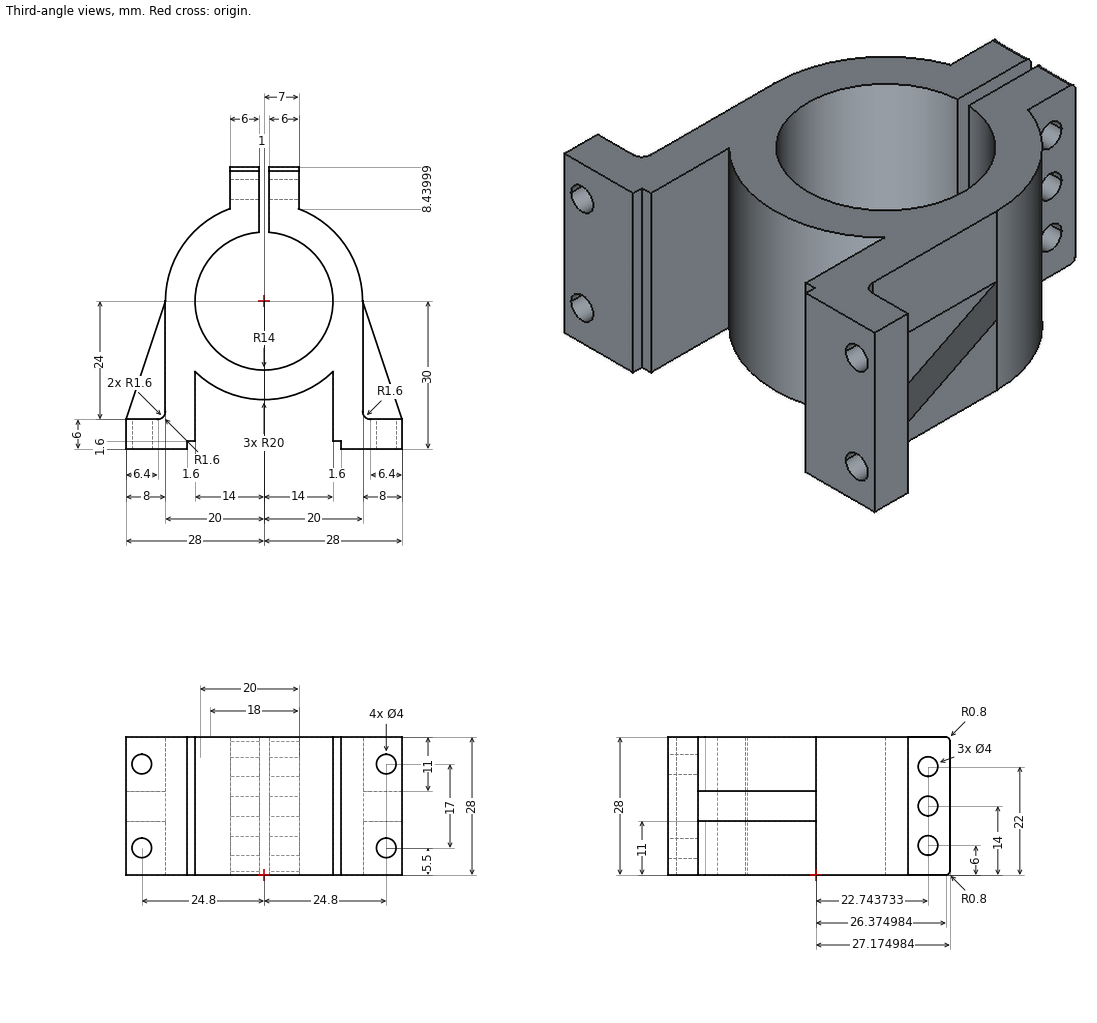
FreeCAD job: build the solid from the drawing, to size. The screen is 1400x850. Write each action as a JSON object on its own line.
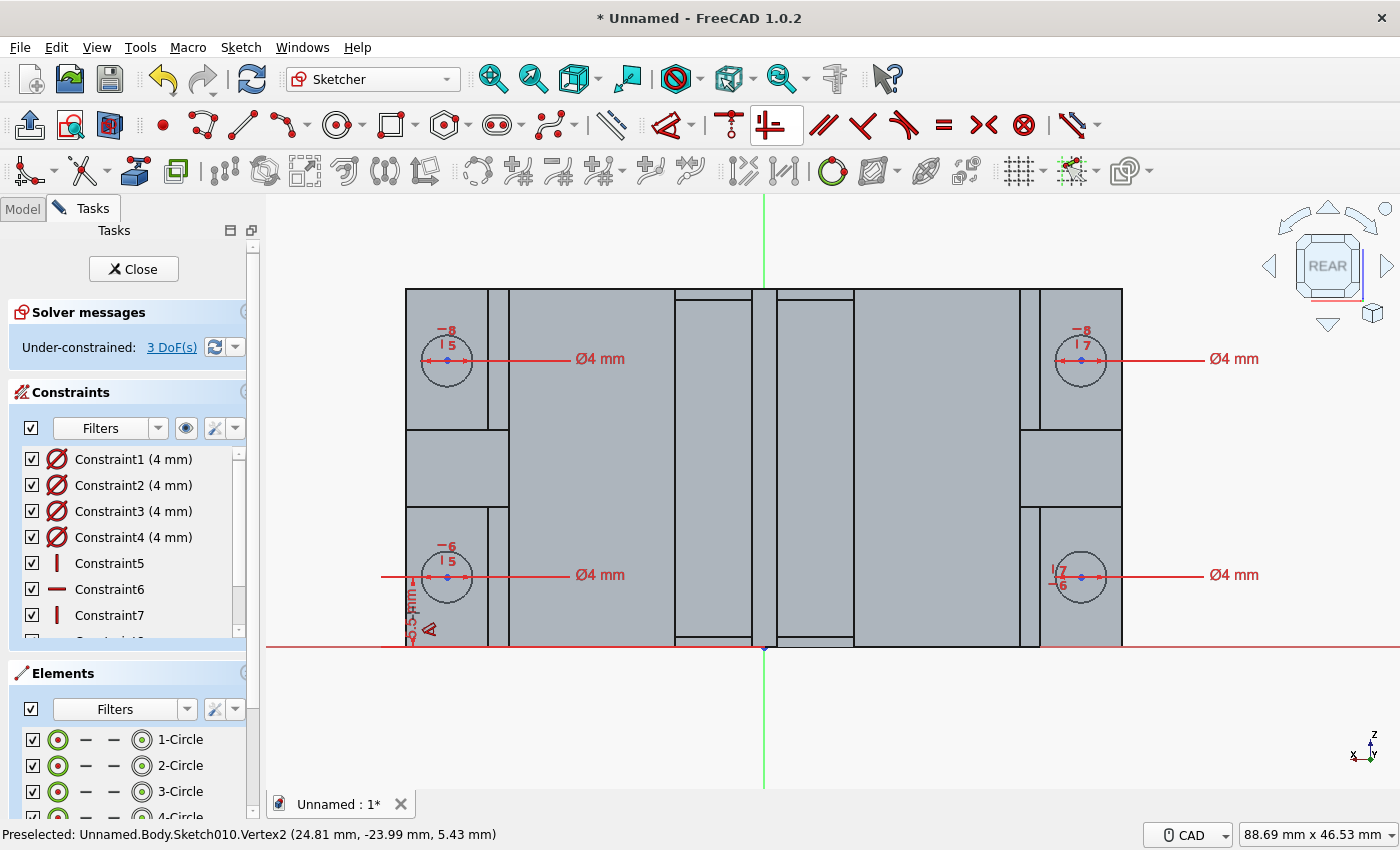
{"action": "left_click", "coordinate": [447, 361]}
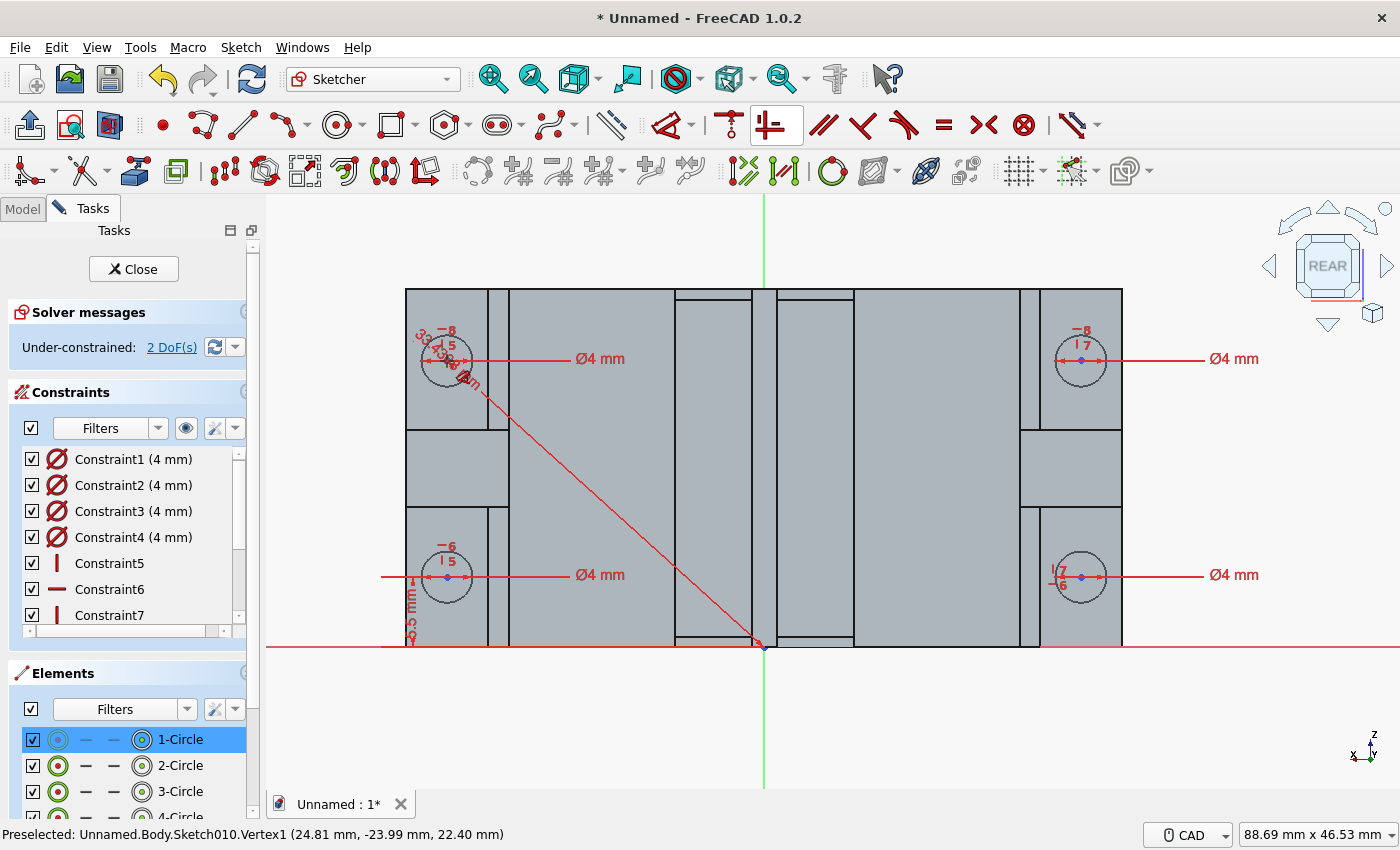
{"action": "left_click", "coordinate": [447, 577]}
{"action": "left_click", "coordinate": [413, 469]}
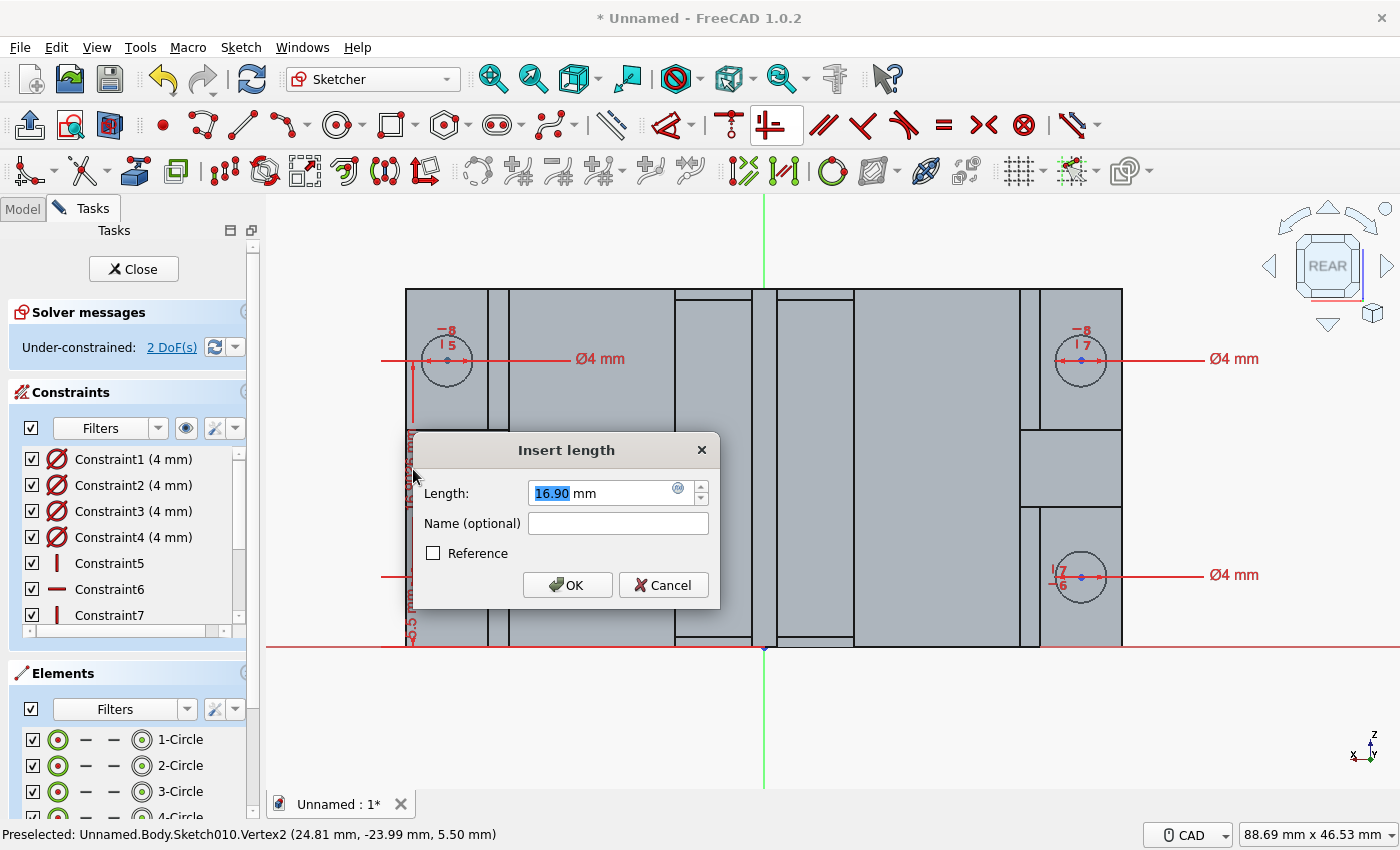
{"action": "type", "text": "17"}
{"action": "key", "text": "Return"}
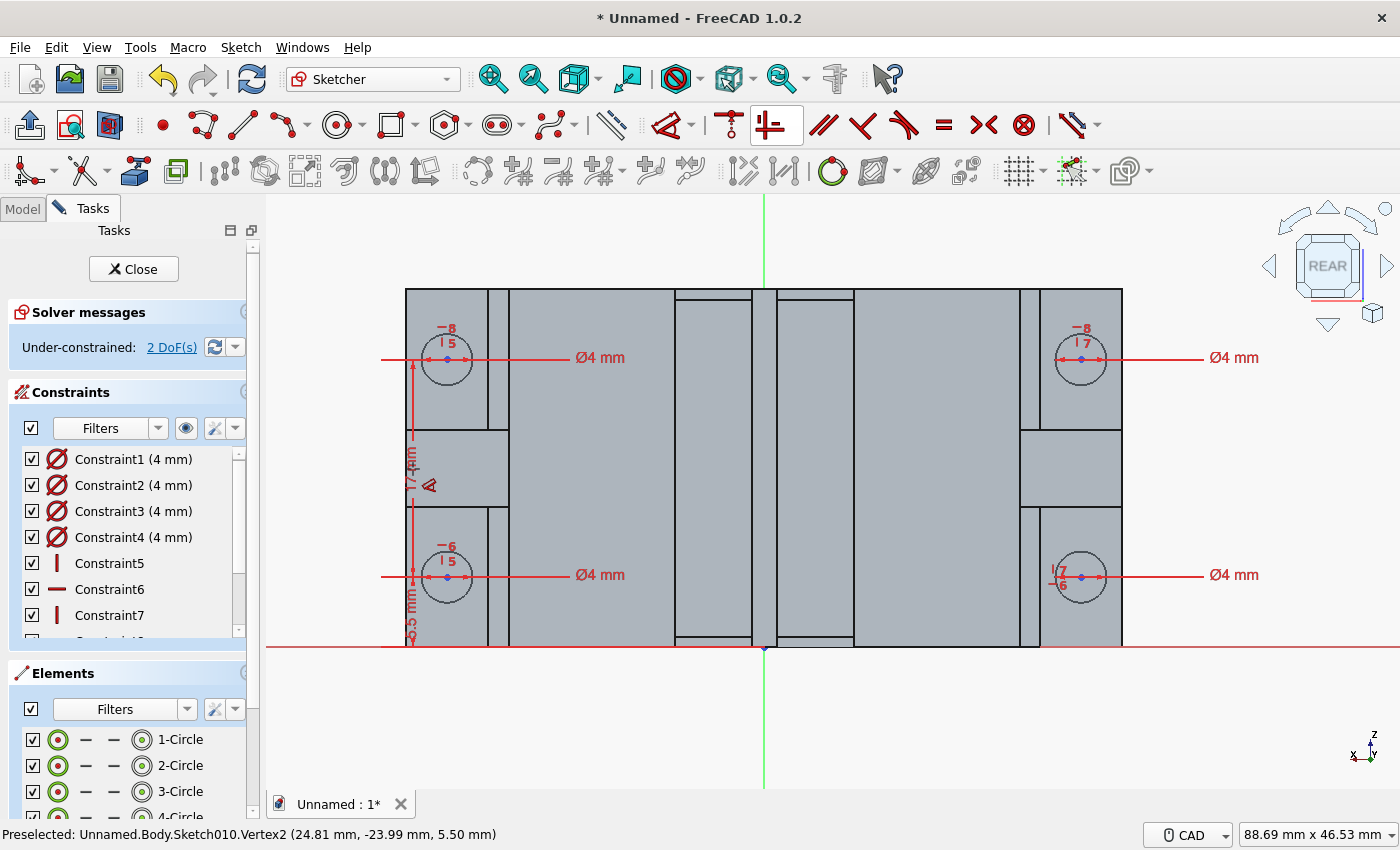
{"action": "left_click", "coordinate": [447, 360]}
{"action": "left_click", "coordinate": [606, 681]}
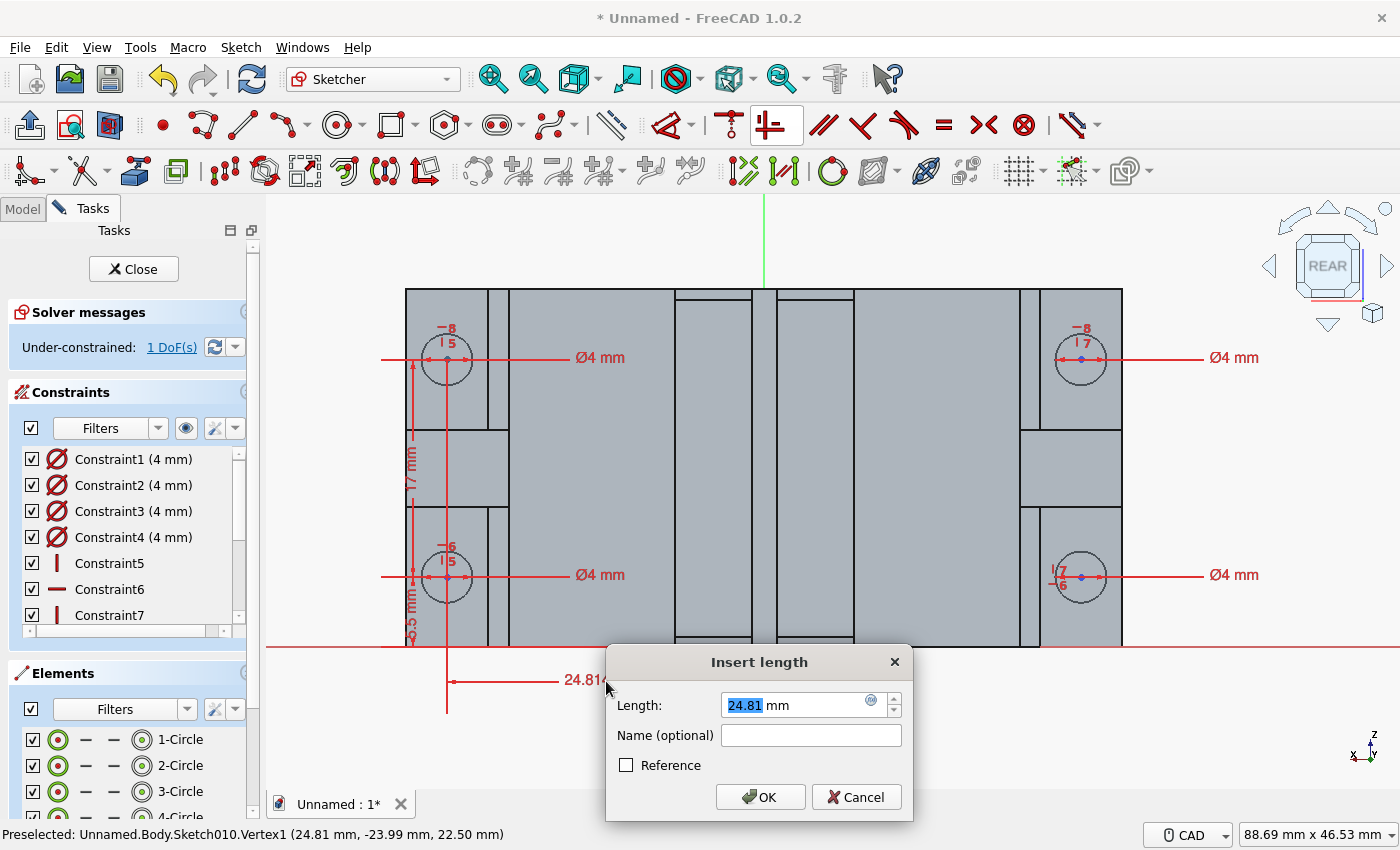
{"action": "type", "text": "24.8"}
{"action": "key", "text": "Return"}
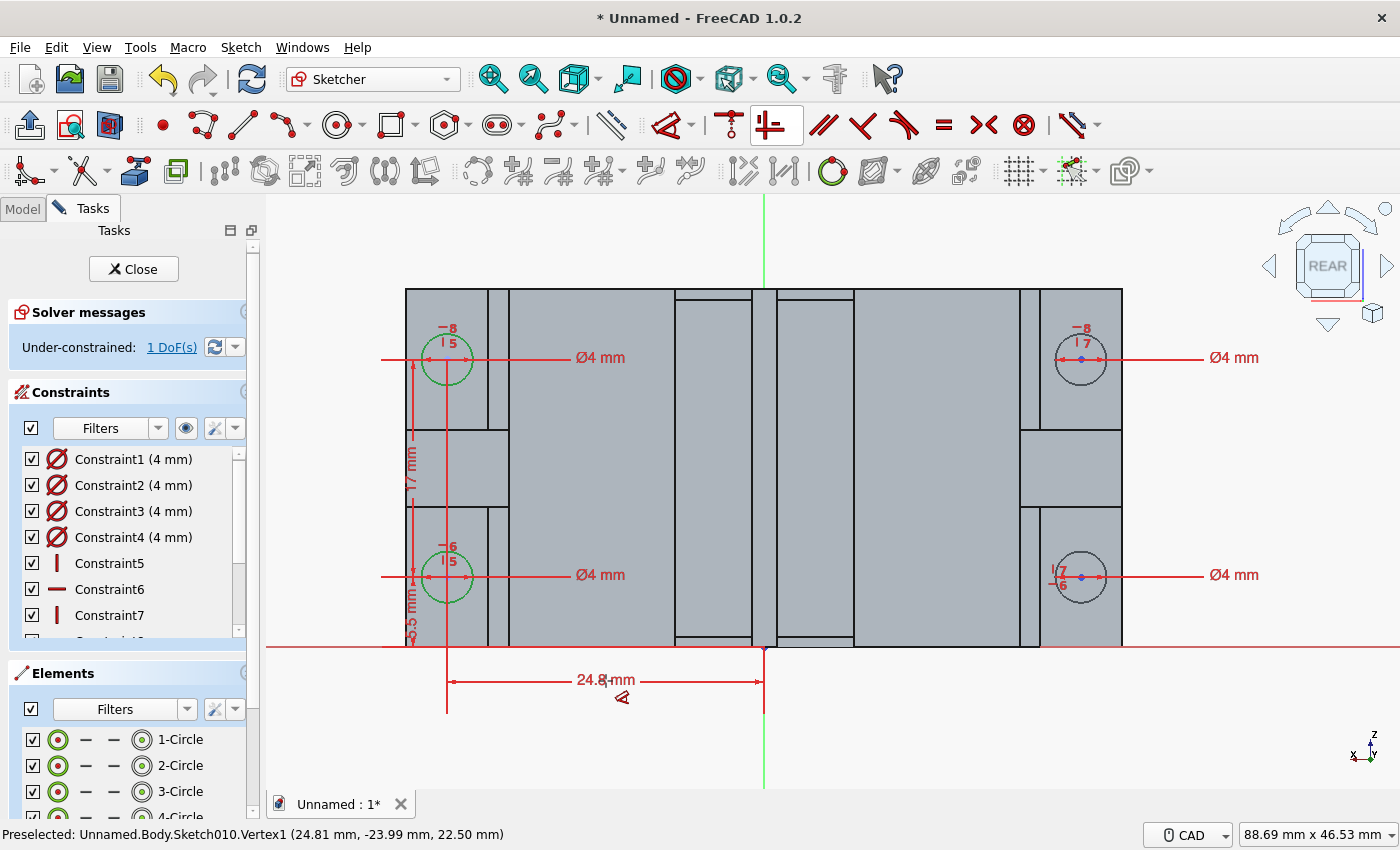
{"action": "left_click", "coordinate": [1081, 577]}
{"action": "left_click", "coordinate": [923, 681]}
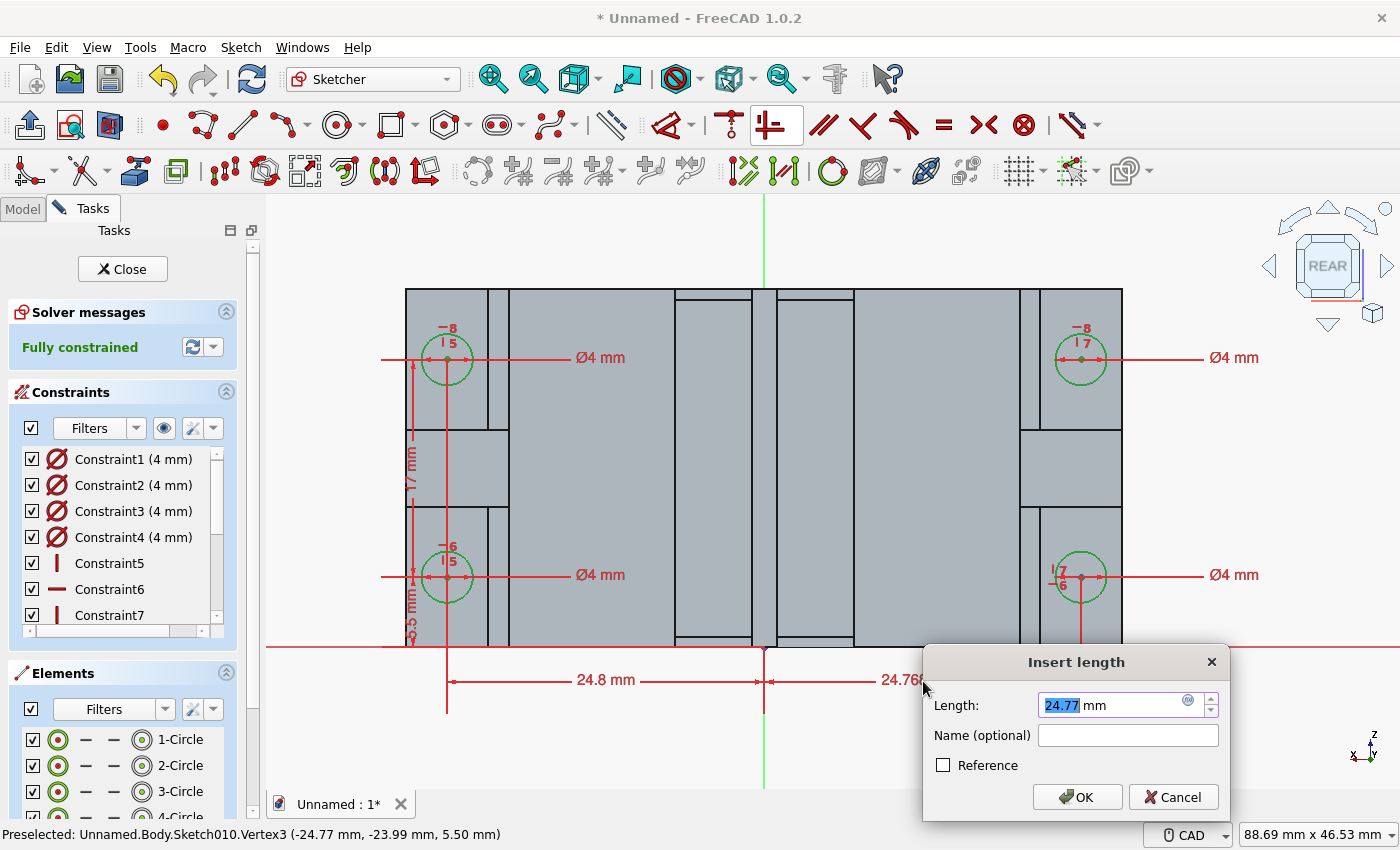
{"action": "type", "text": "24.8"}
{"action": "key", "text": "Return"}
{"action": "key", "text": "Escape"}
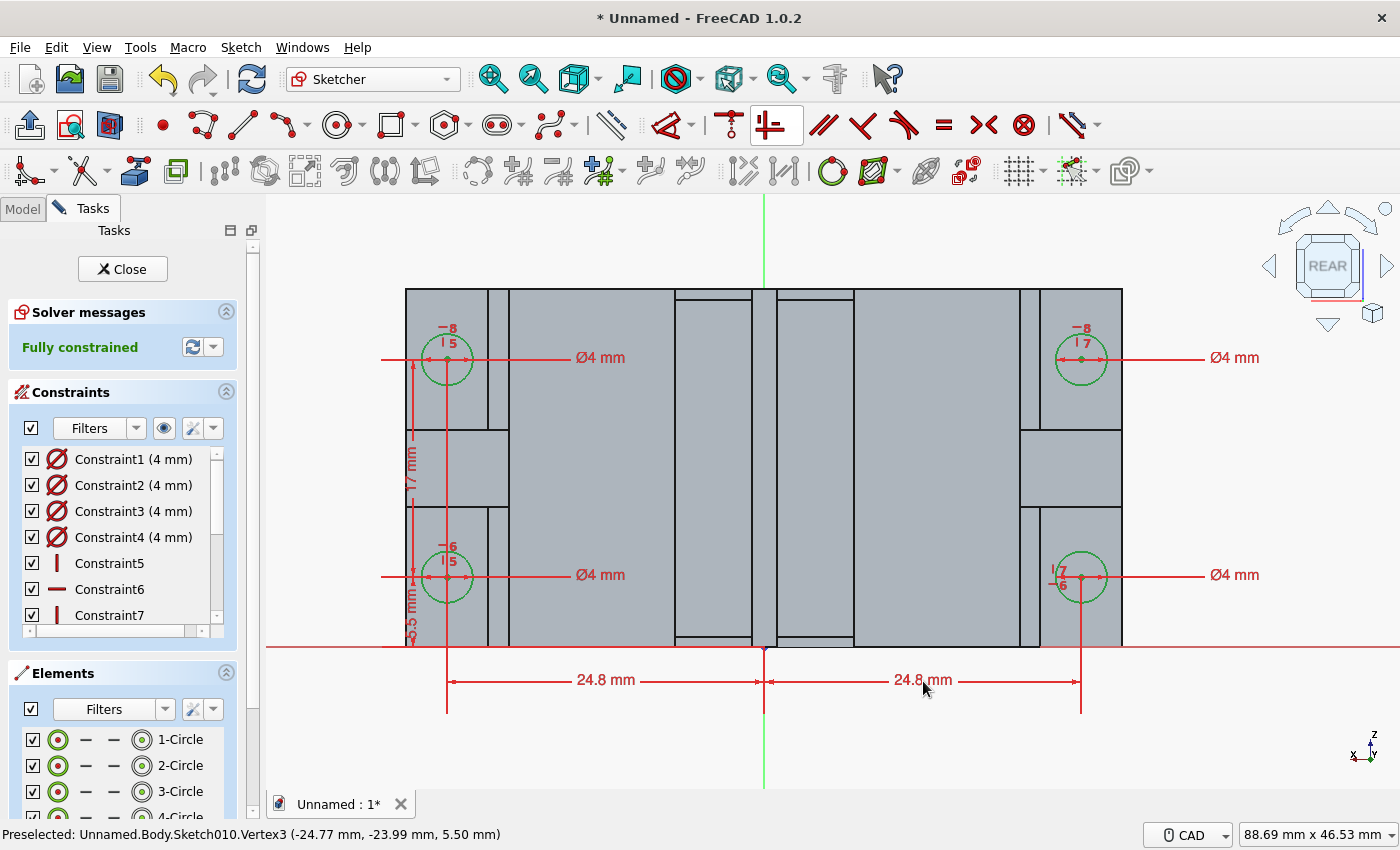
{"action": "left_click", "coordinate": [123, 269]}